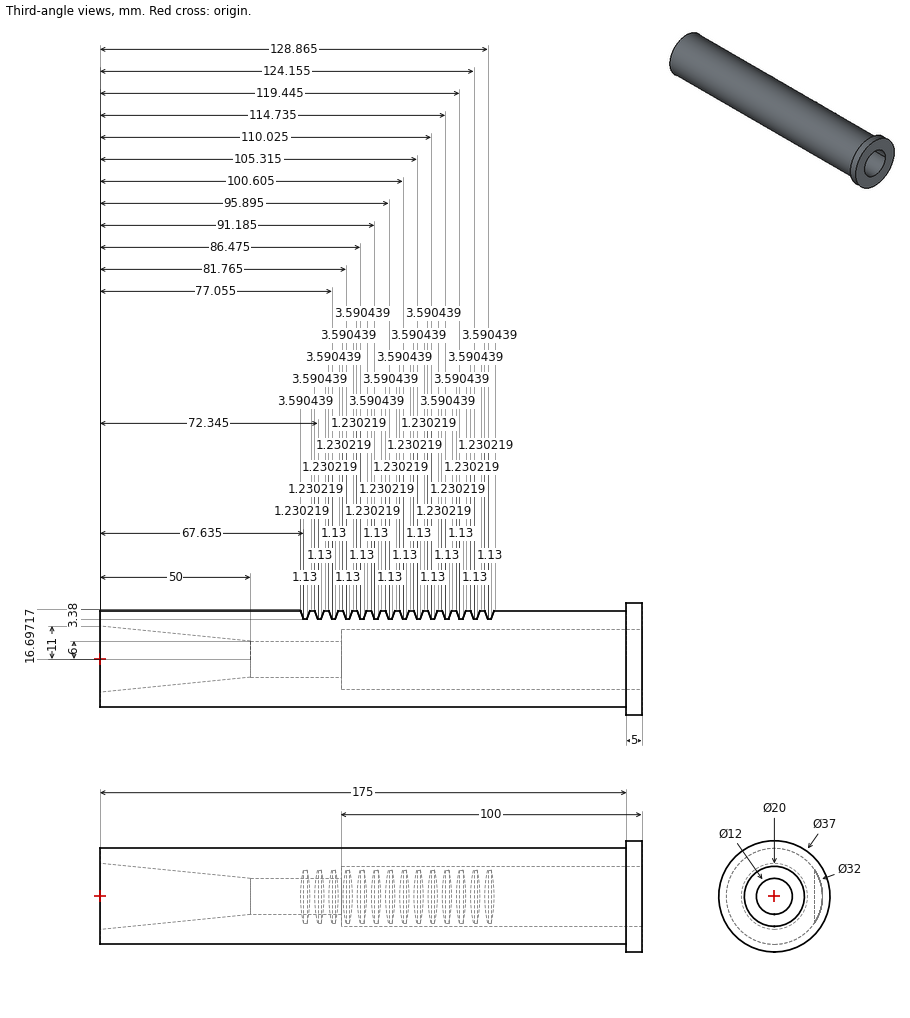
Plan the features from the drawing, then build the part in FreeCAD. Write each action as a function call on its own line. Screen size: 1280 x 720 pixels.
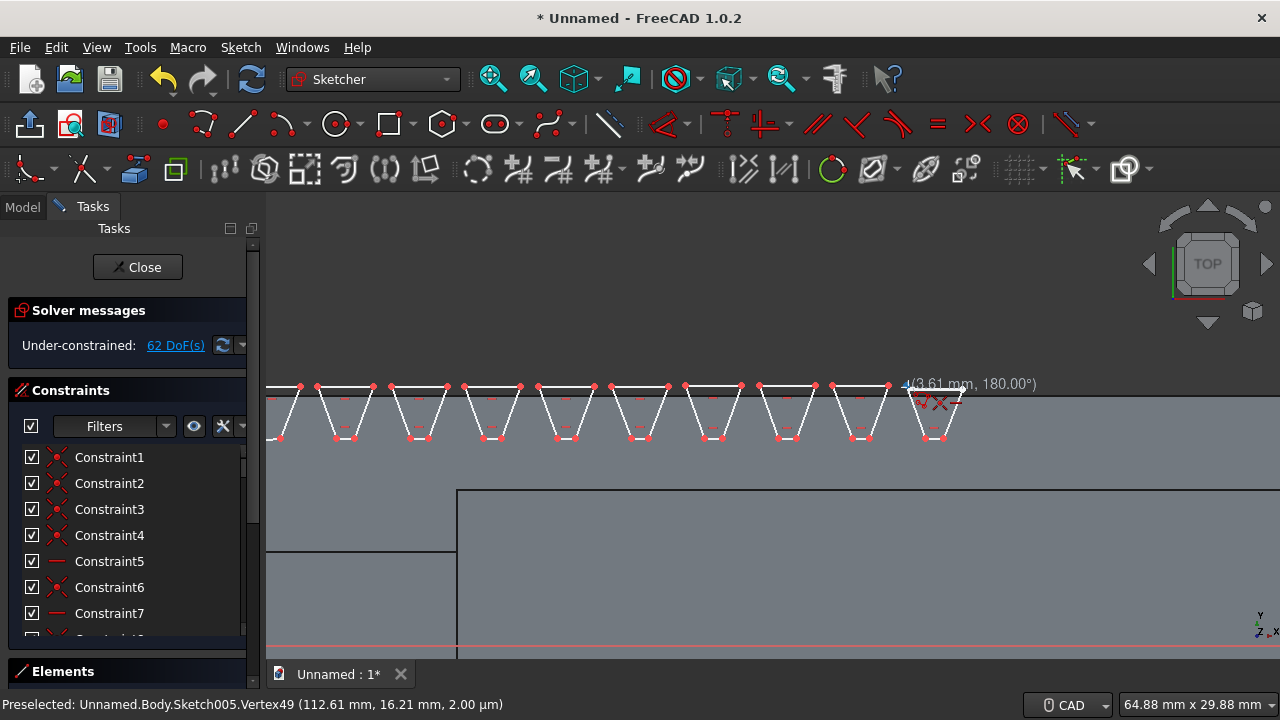
click(907, 386)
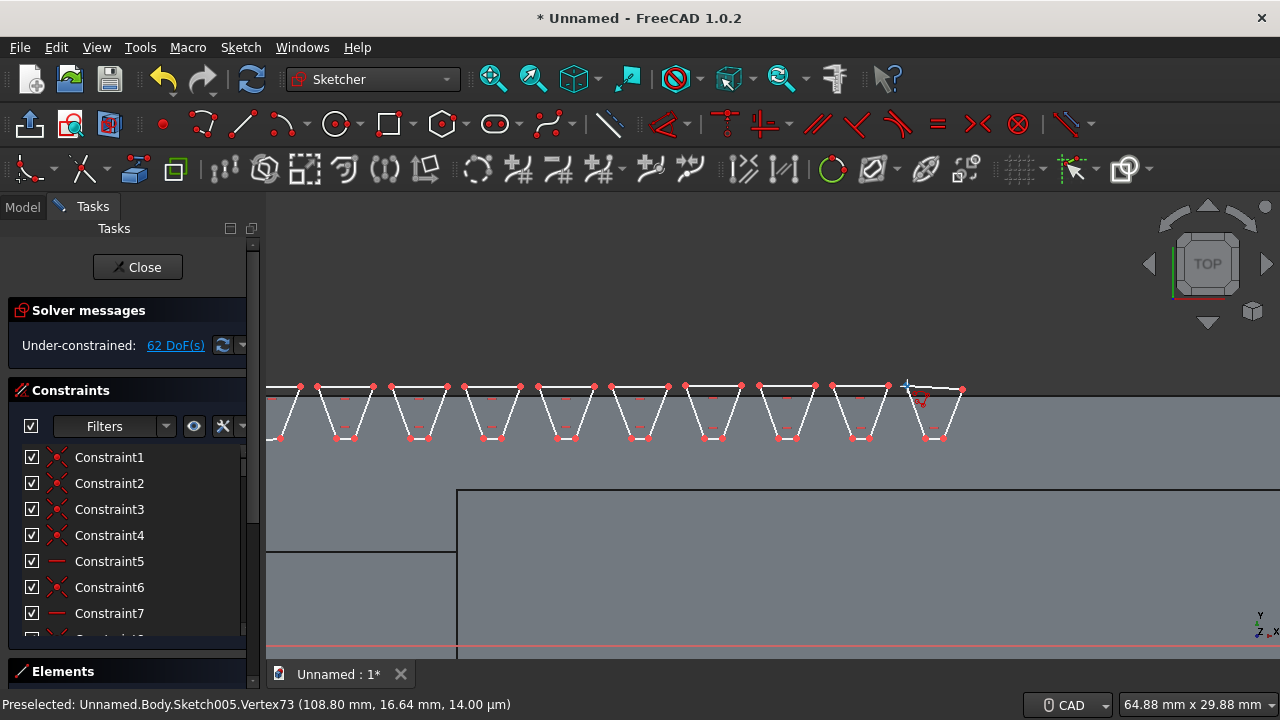
click(980, 385)
click(1000, 438)
click(1017, 438)
click(1036, 385)
click(980, 386)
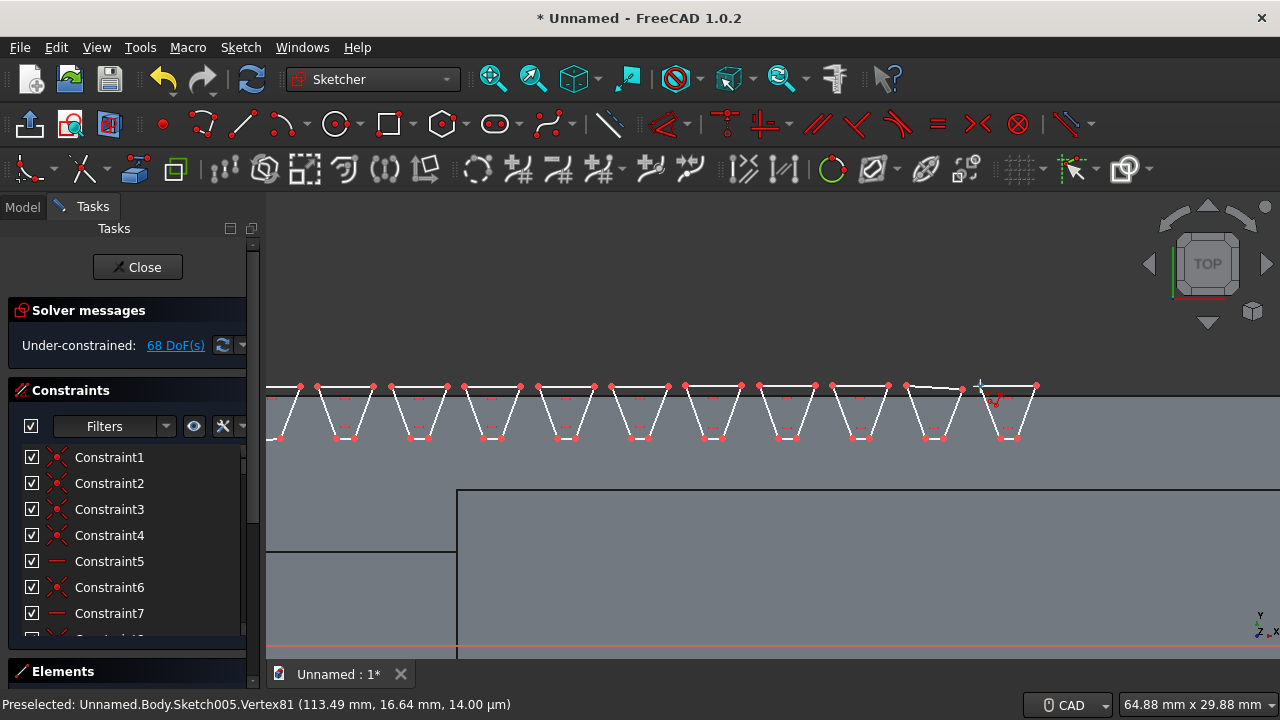
click(1054, 385)
click(1073, 438)
click(1091, 438)
click(1110, 385)
click(1054, 386)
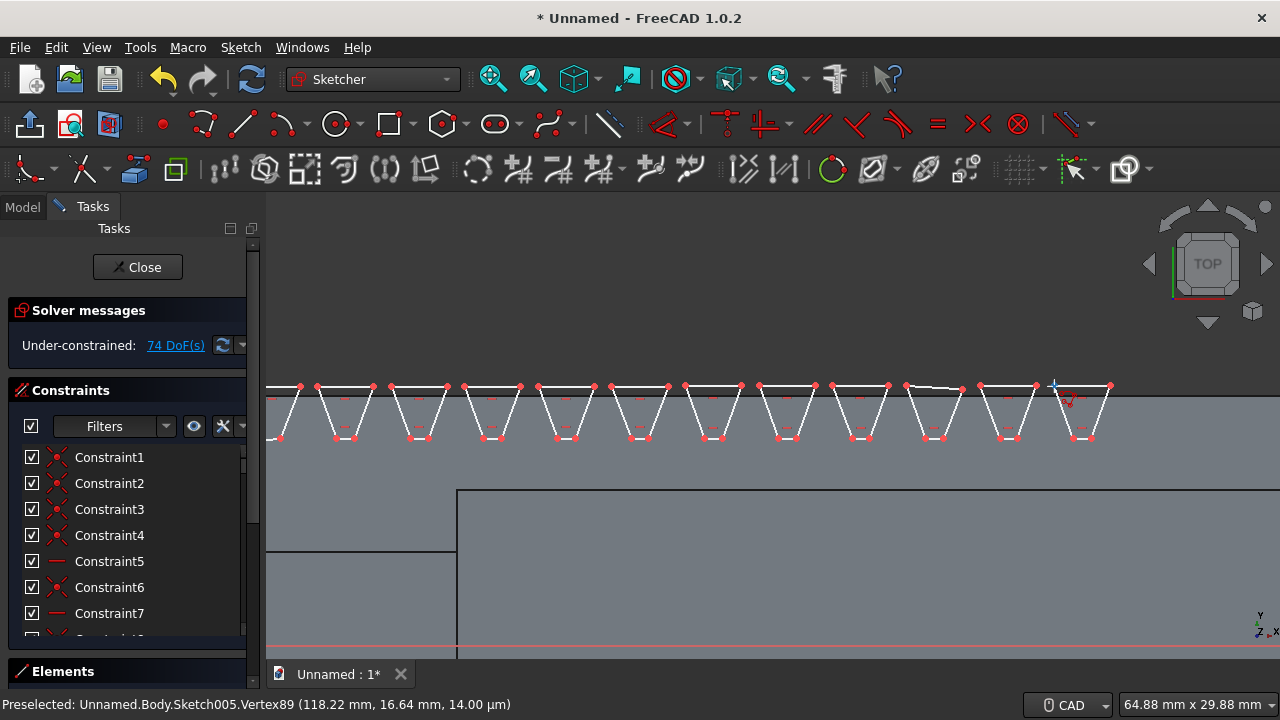
scroll(908, 387, down, 6)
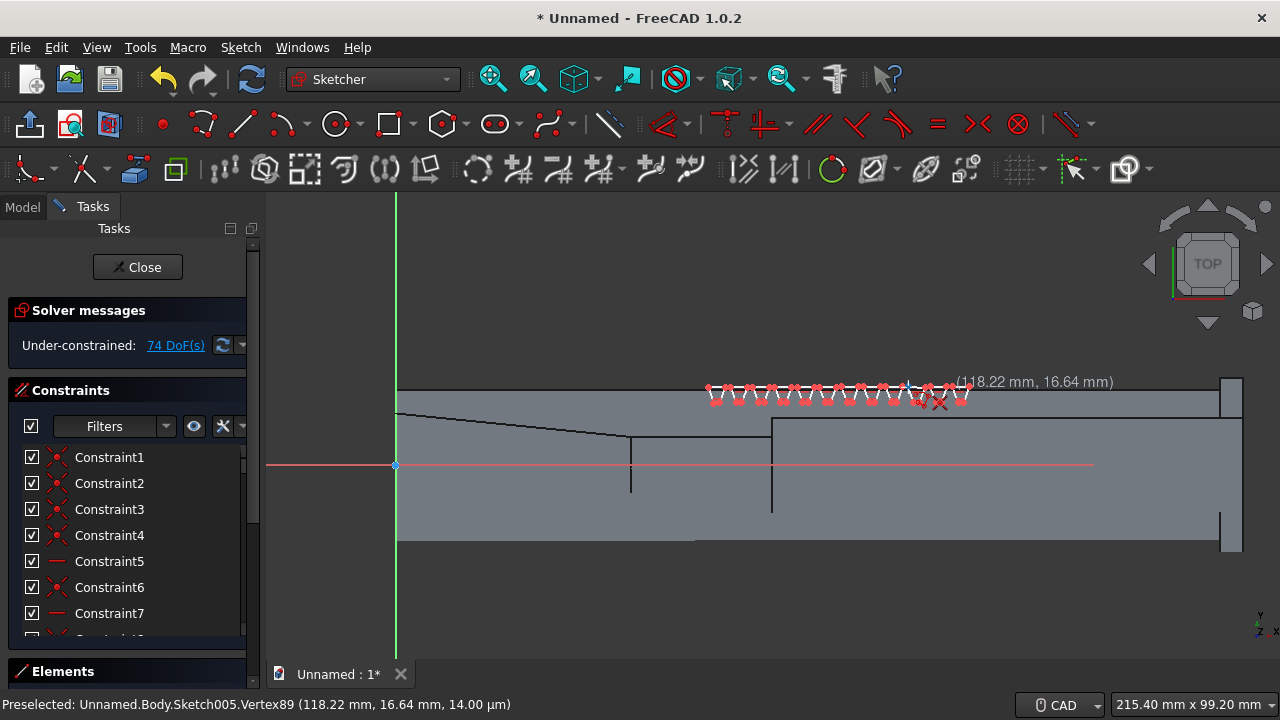
scroll(975, 387, up, 6)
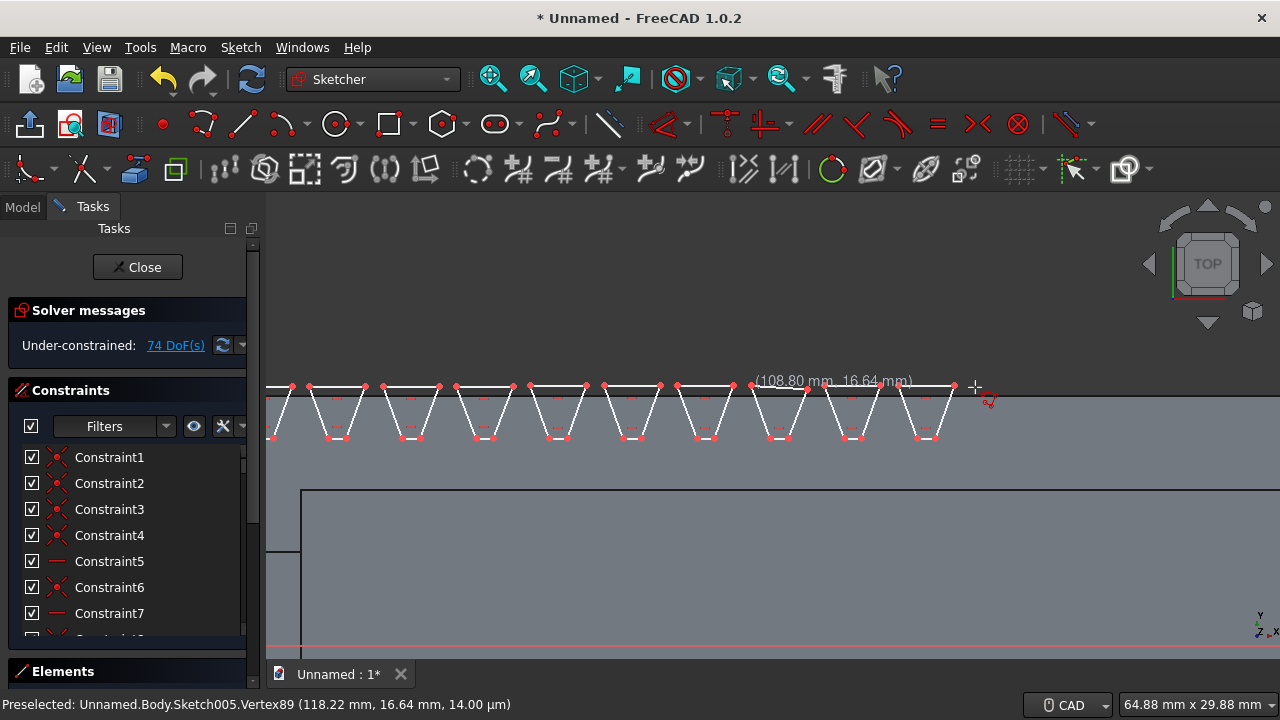
click(972, 385)
click(991, 438)
click(1009, 438)
click(1028, 385)
click(972, 386)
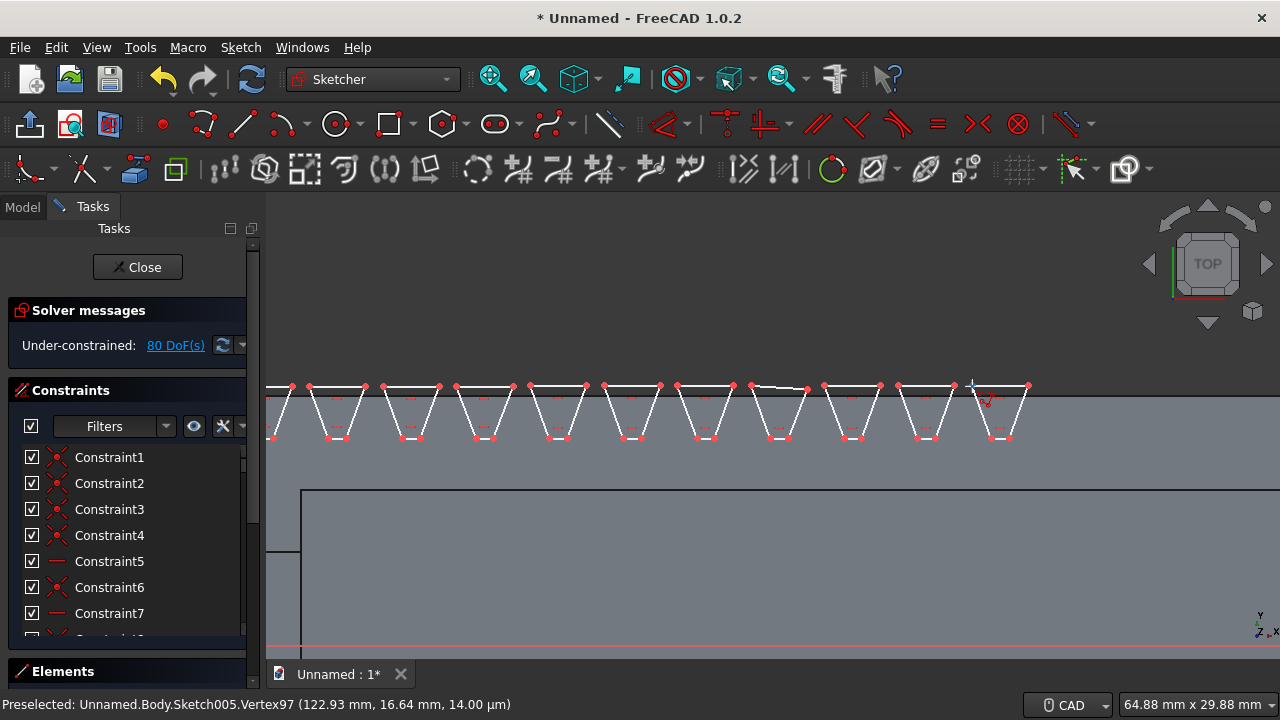
click(1046, 385)
click(1065, 438)
click(1082, 438)
click(1102, 385)
click(1046, 386)
key(Escape)
key(Escape)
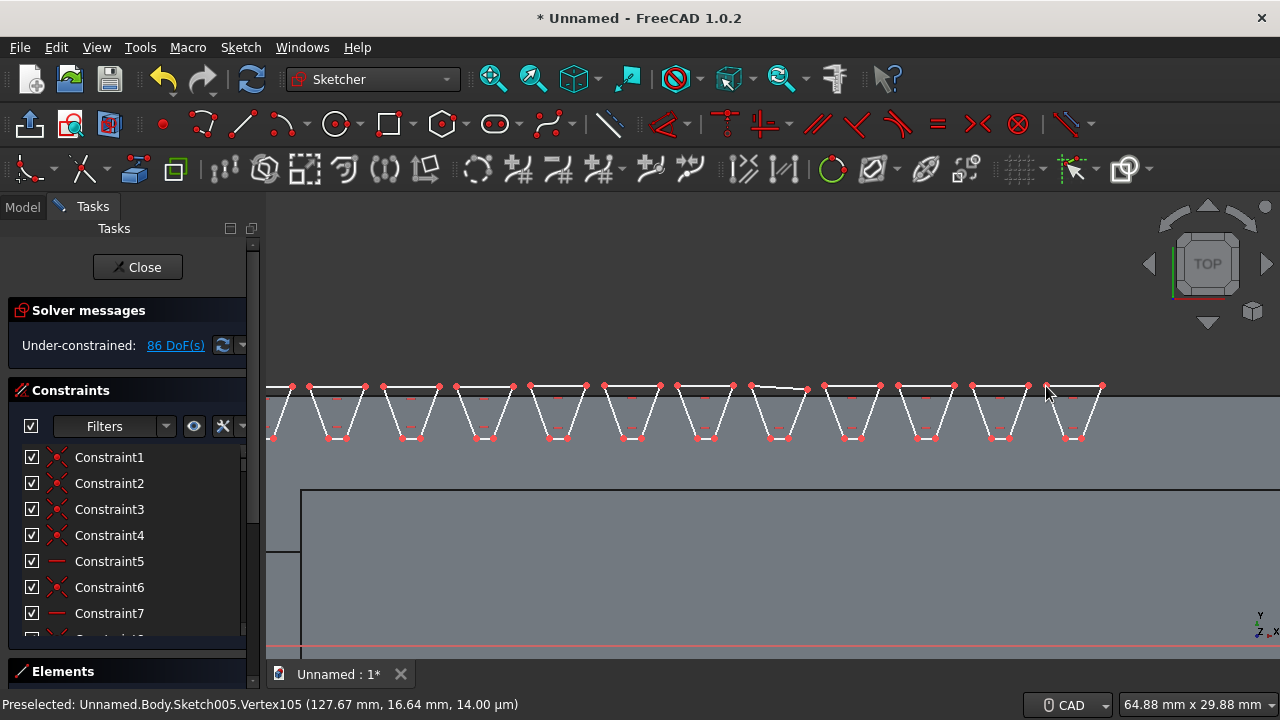
scroll(975, 387, down, 6)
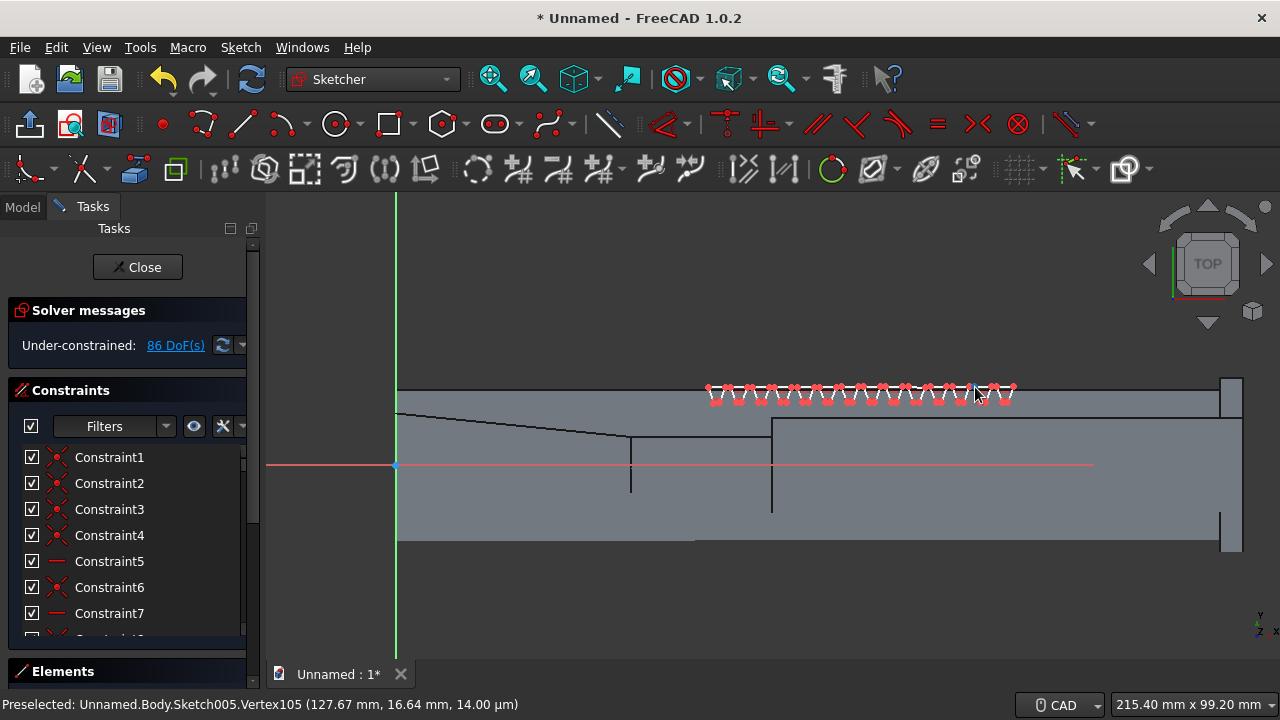
scroll(717, 403, up, 8)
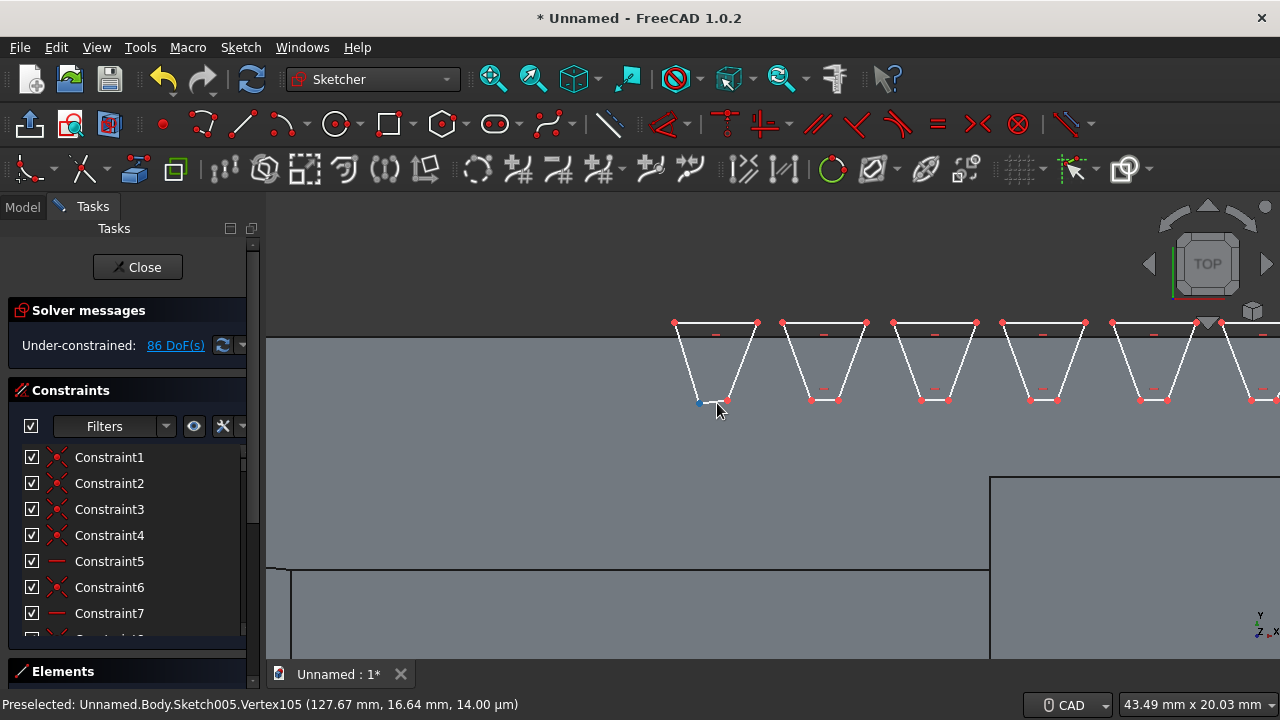
click(714, 402)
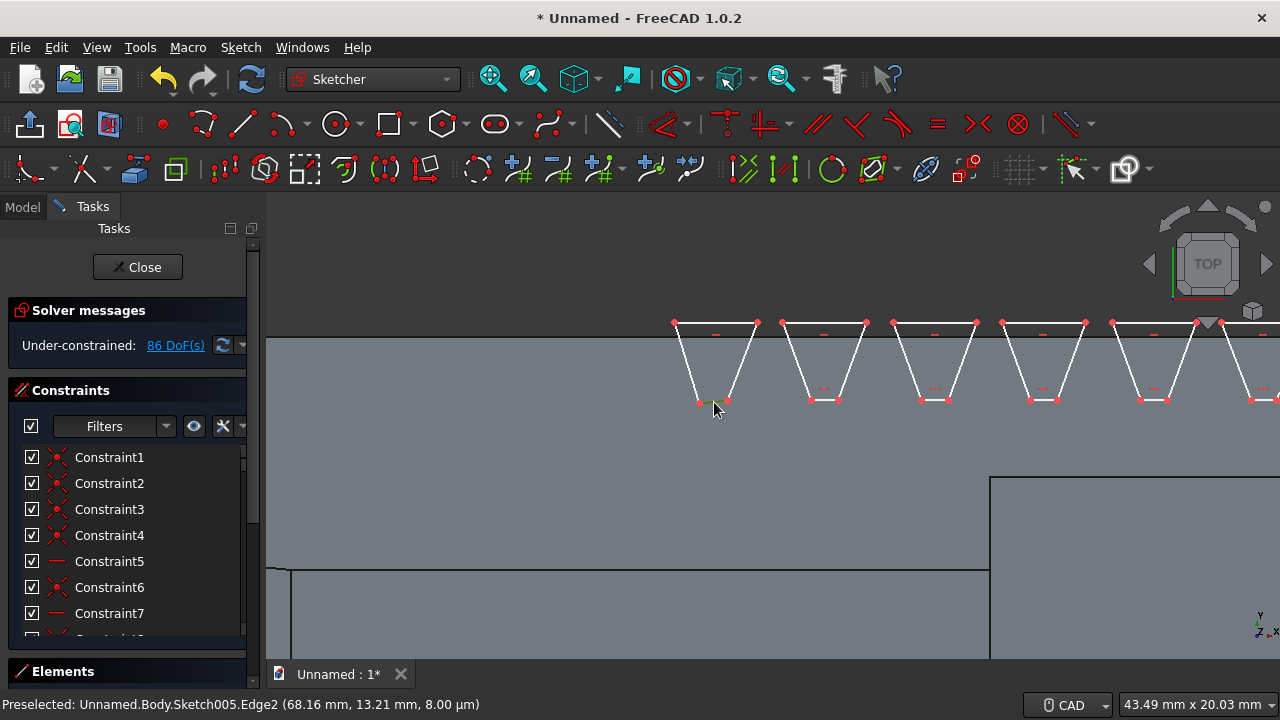
key(h)